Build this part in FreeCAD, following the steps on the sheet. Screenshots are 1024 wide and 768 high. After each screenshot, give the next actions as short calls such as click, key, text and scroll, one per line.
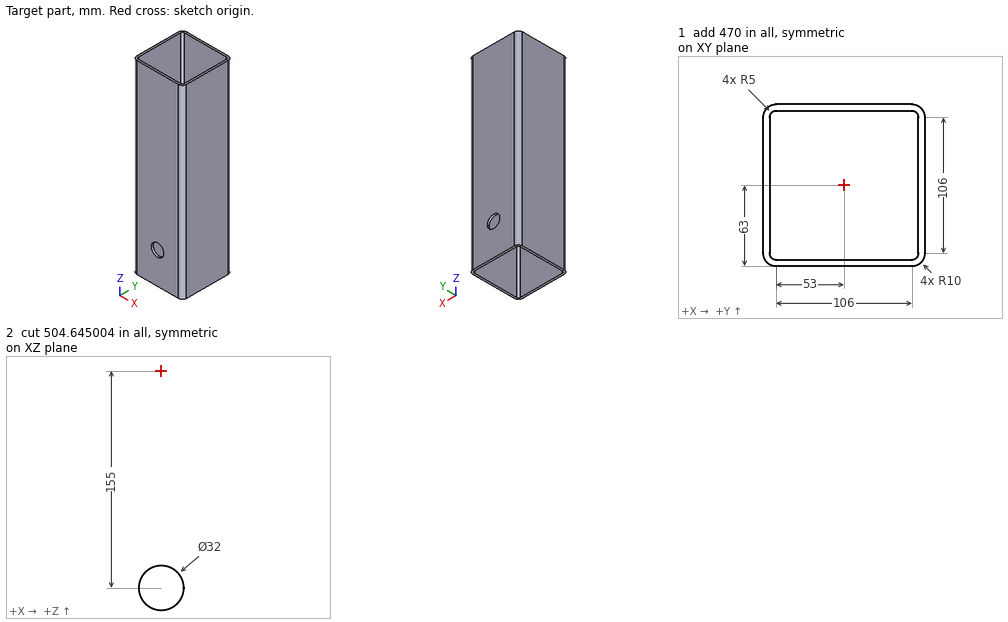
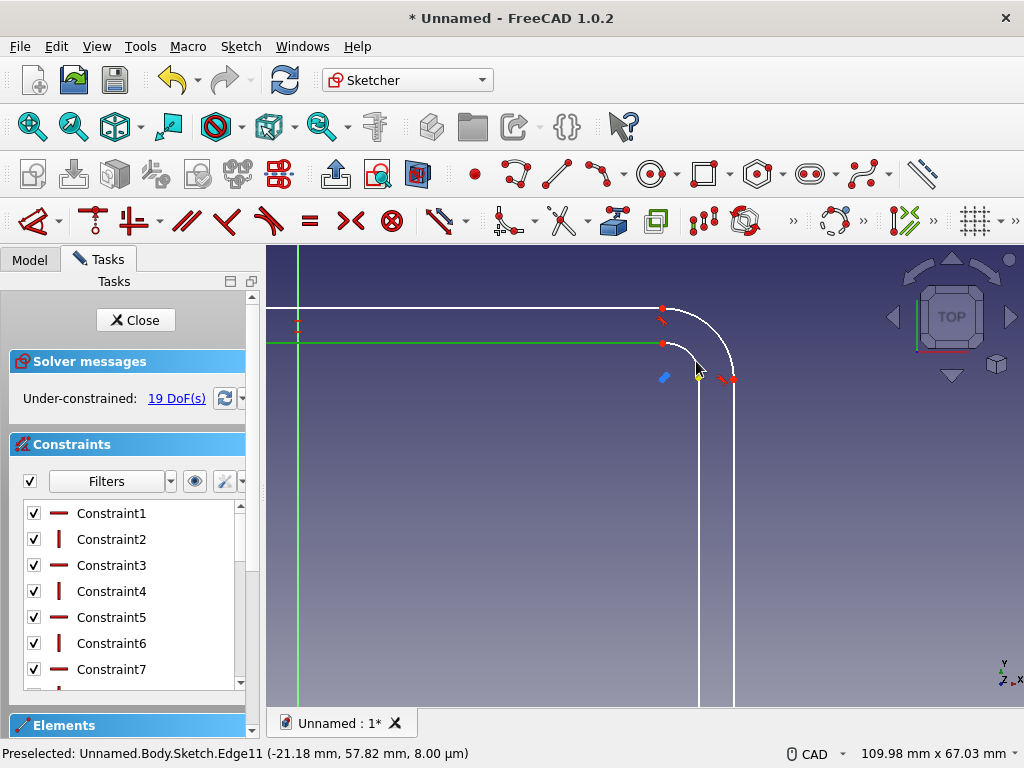
click(695, 361)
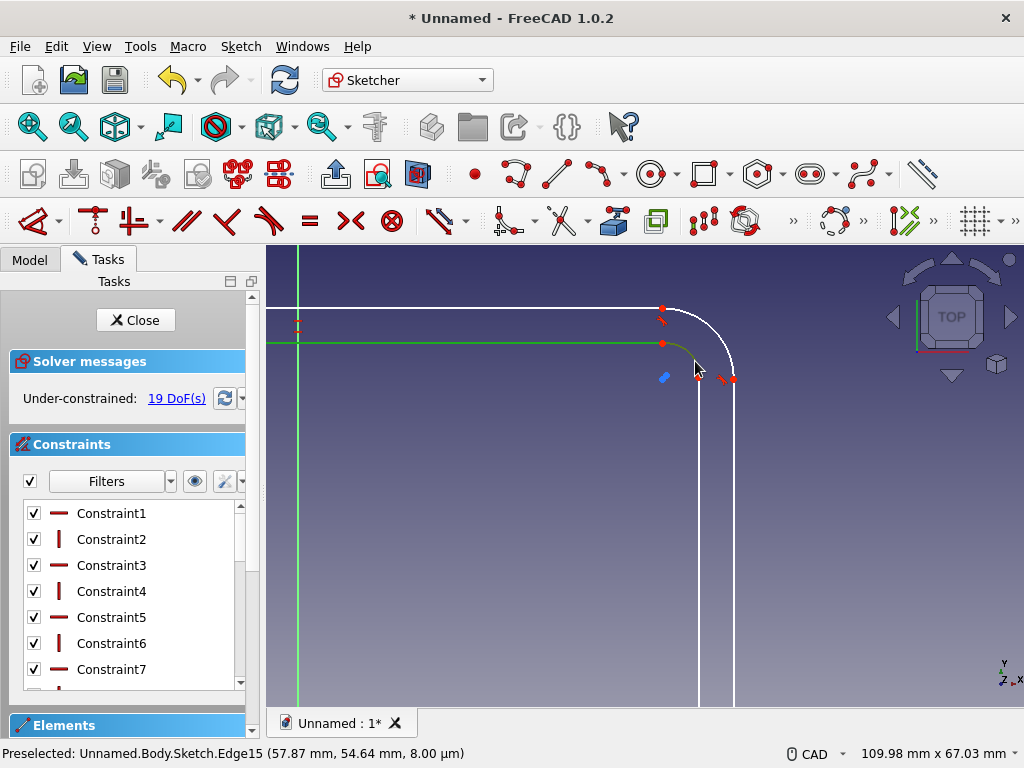
click(269, 222)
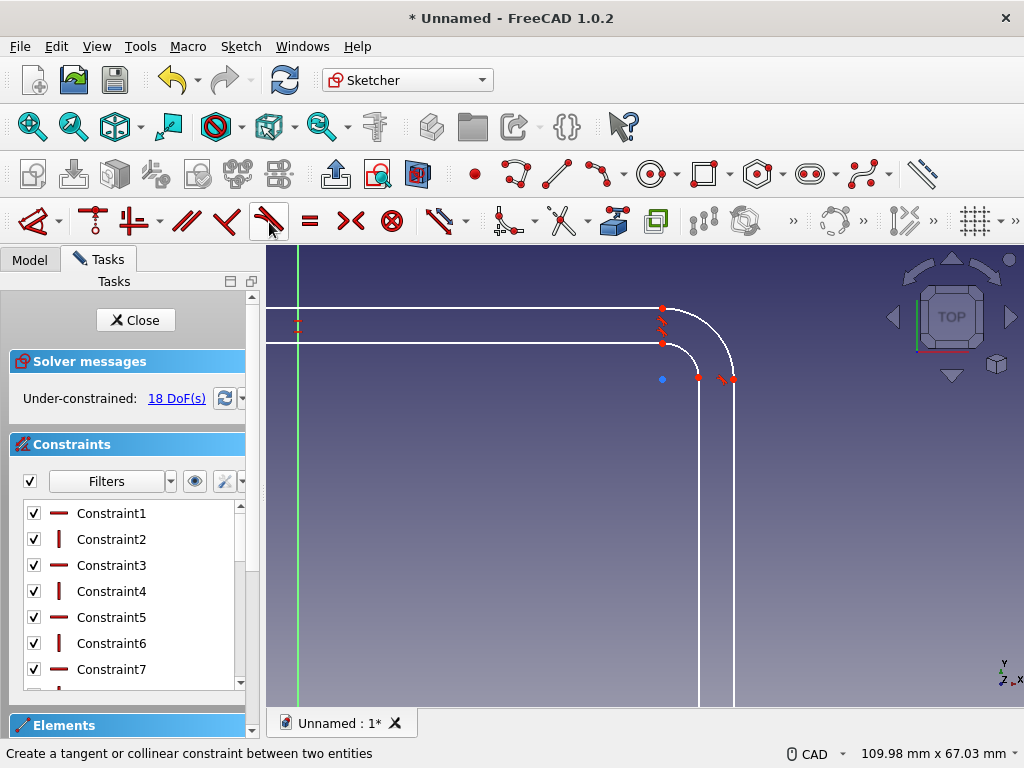
click(699, 597)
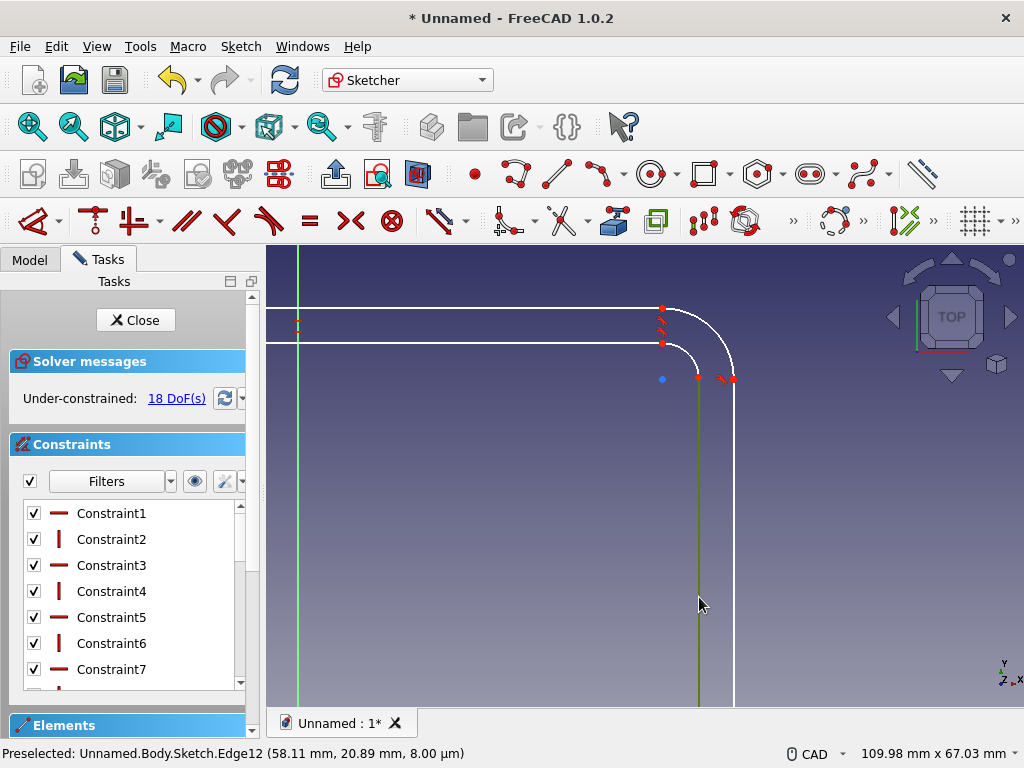
click(694, 362)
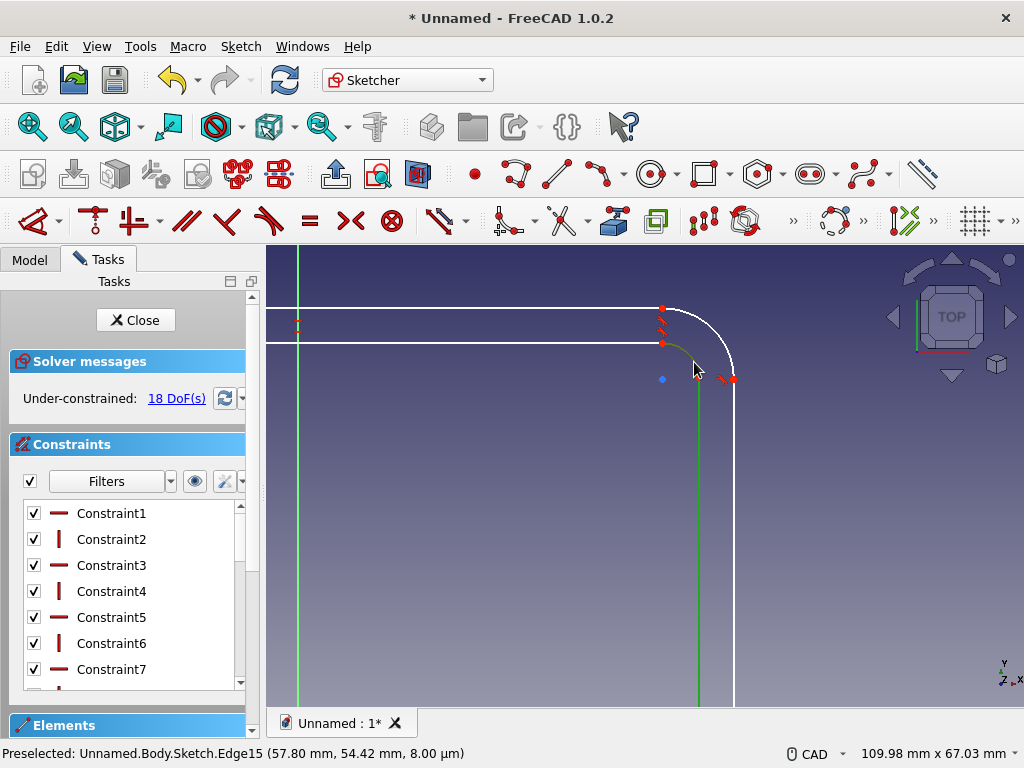
click(269, 222)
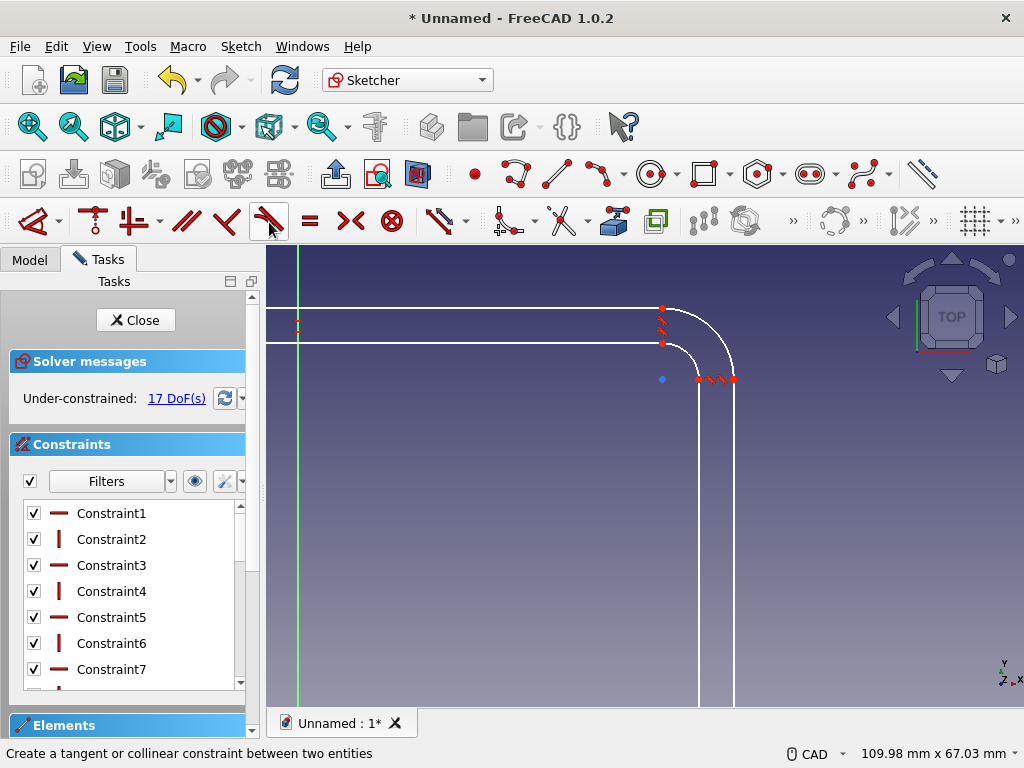
click(699, 598)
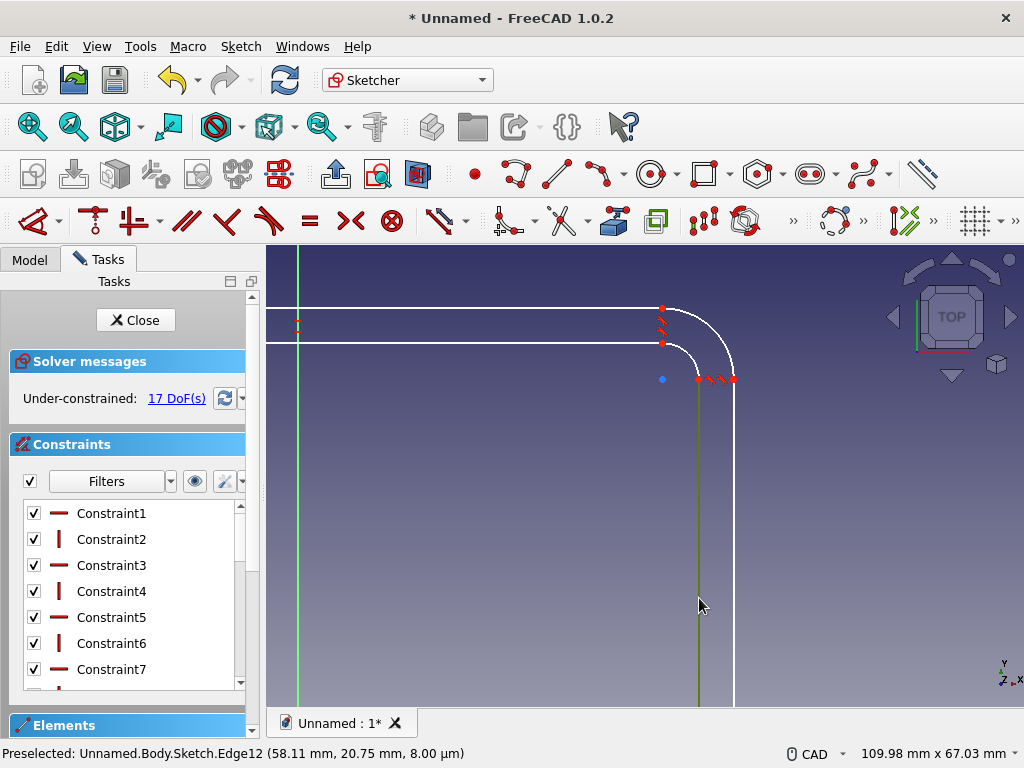
scroll(696, 361, down, 6)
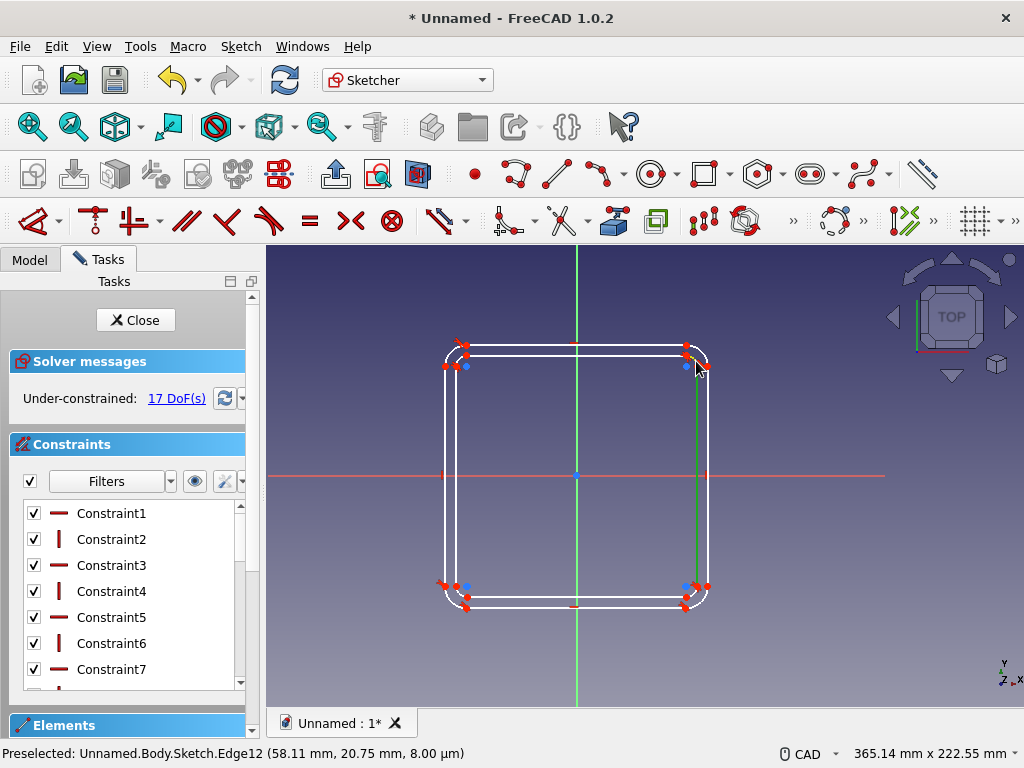
scroll(691, 596, up, 6)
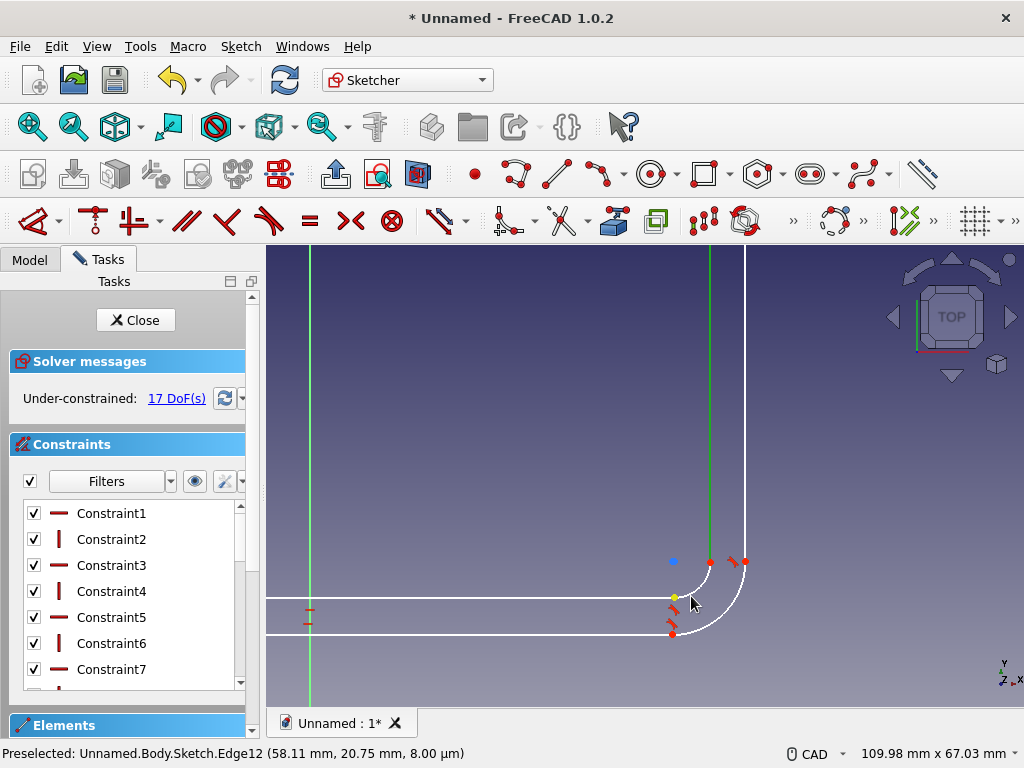
click(690, 594)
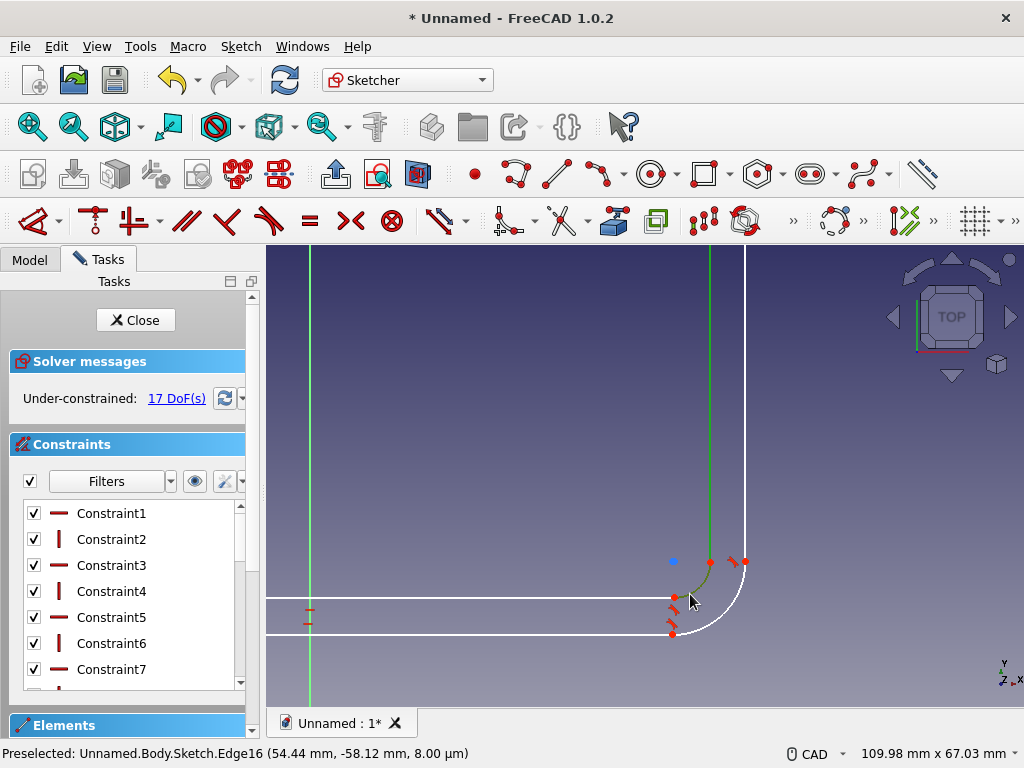
click(269, 222)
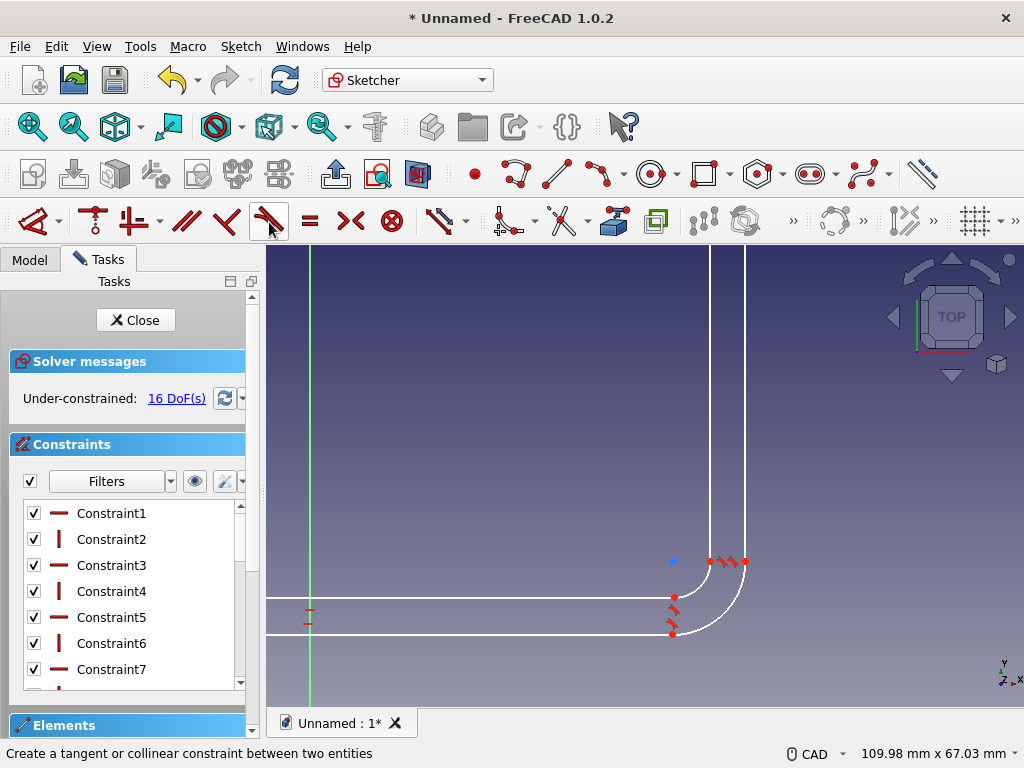
scroll(691, 597, down, 6)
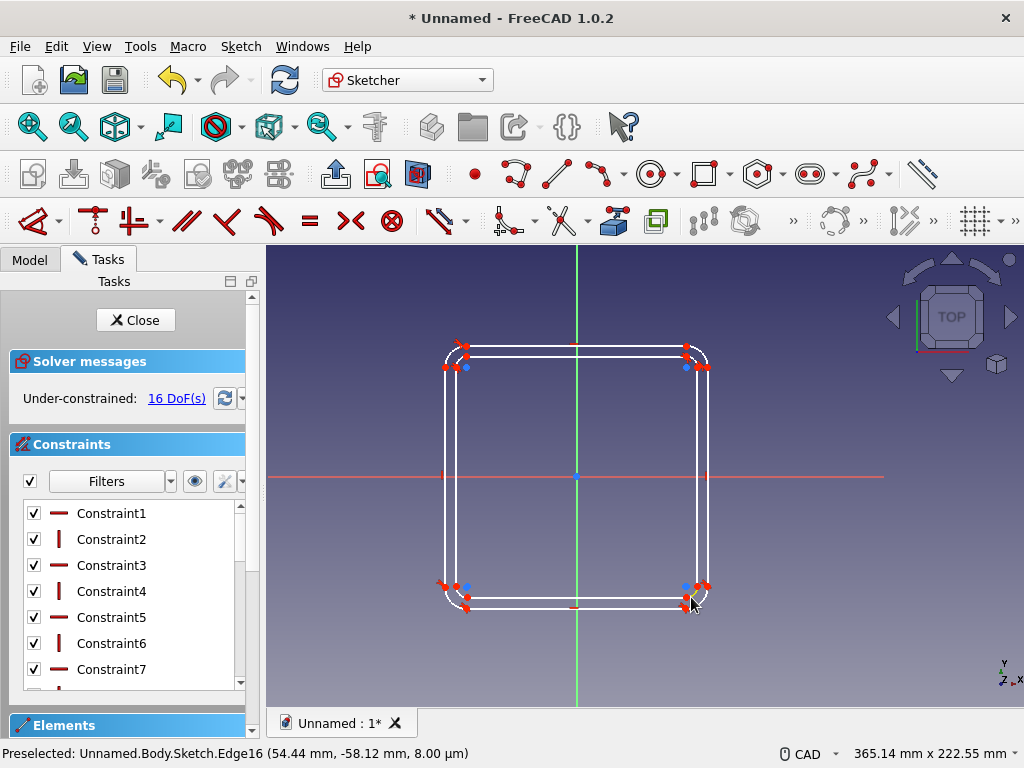
scroll(447, 597, up, 2)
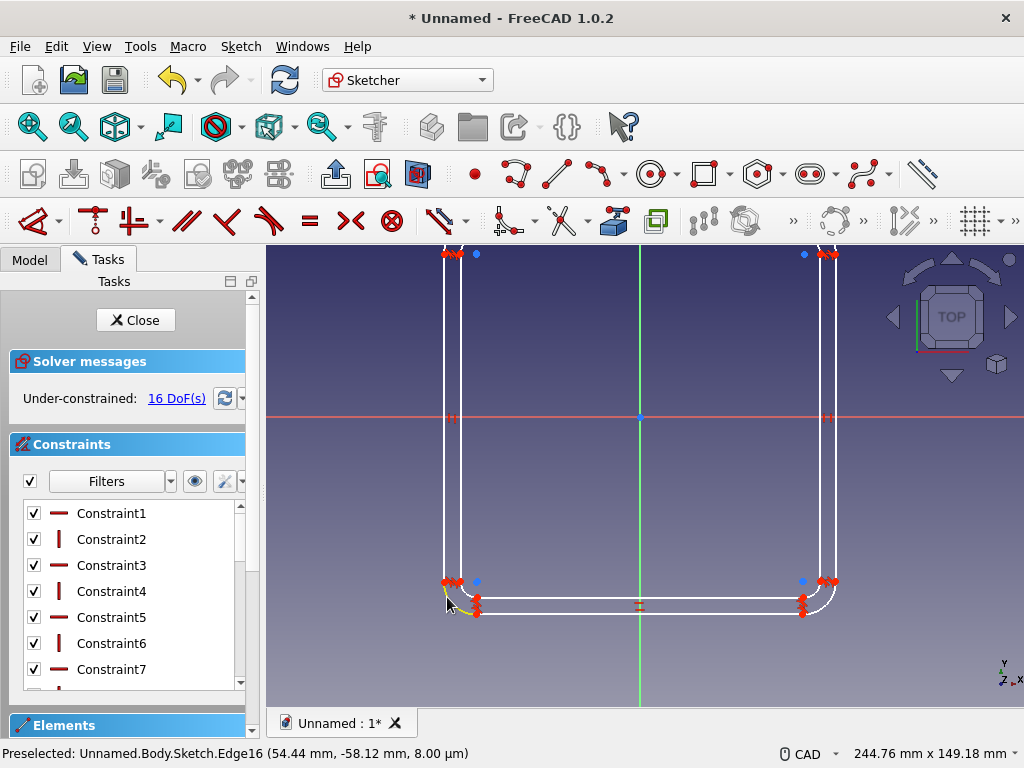
click(448, 597)